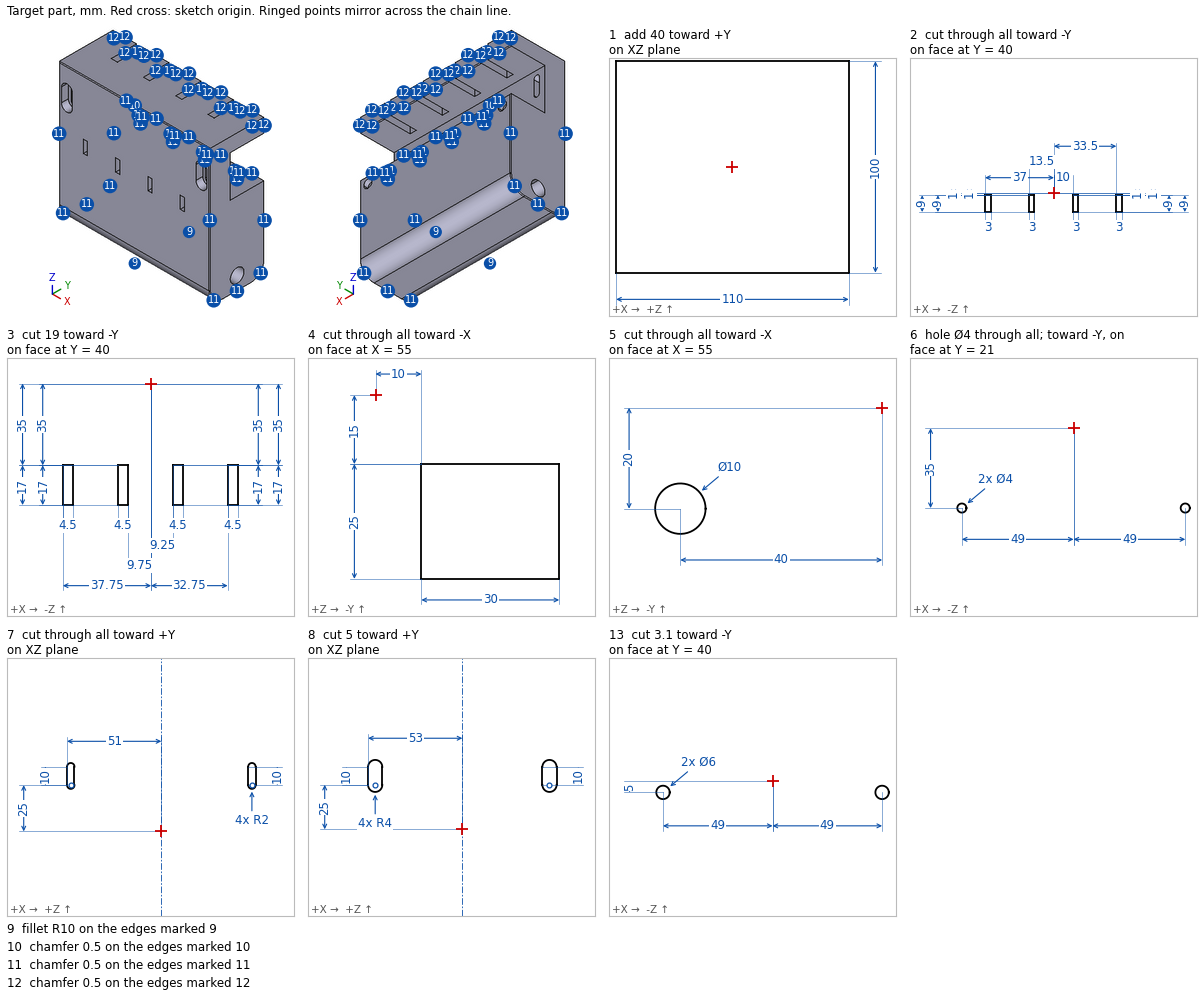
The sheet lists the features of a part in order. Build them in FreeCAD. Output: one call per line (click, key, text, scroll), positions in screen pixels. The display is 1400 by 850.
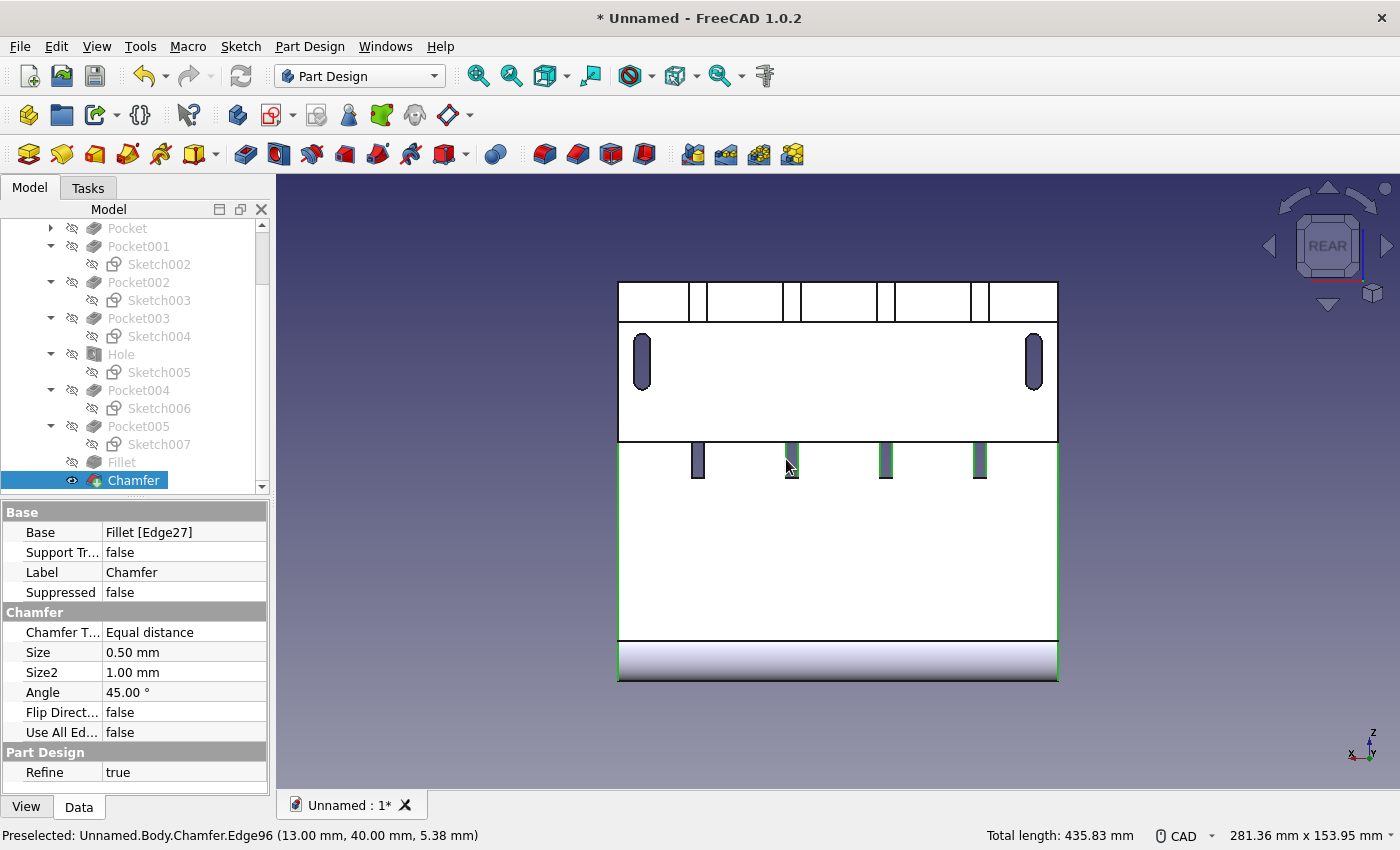
click(704, 459, ctrl)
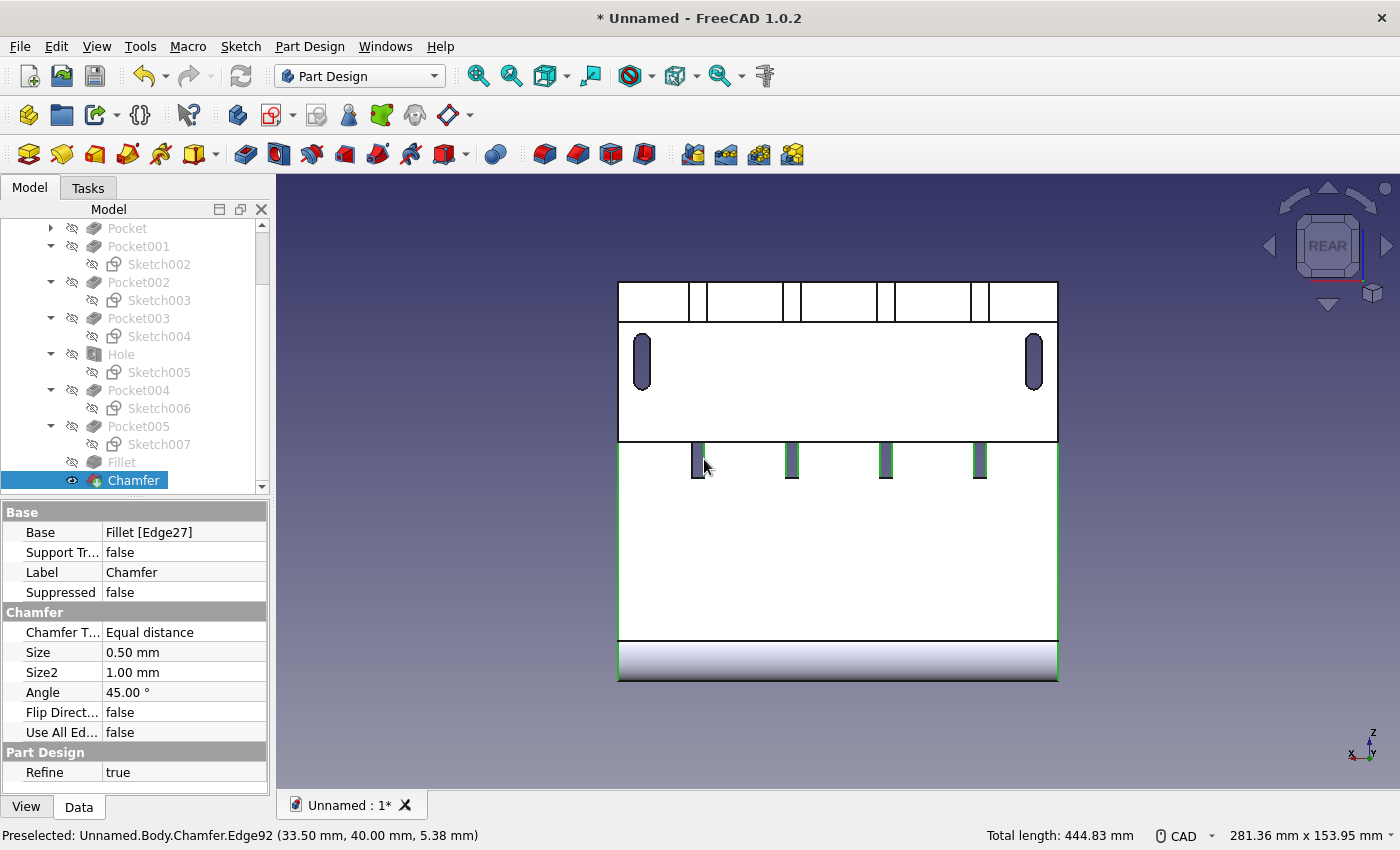
click(692, 459, ctrl)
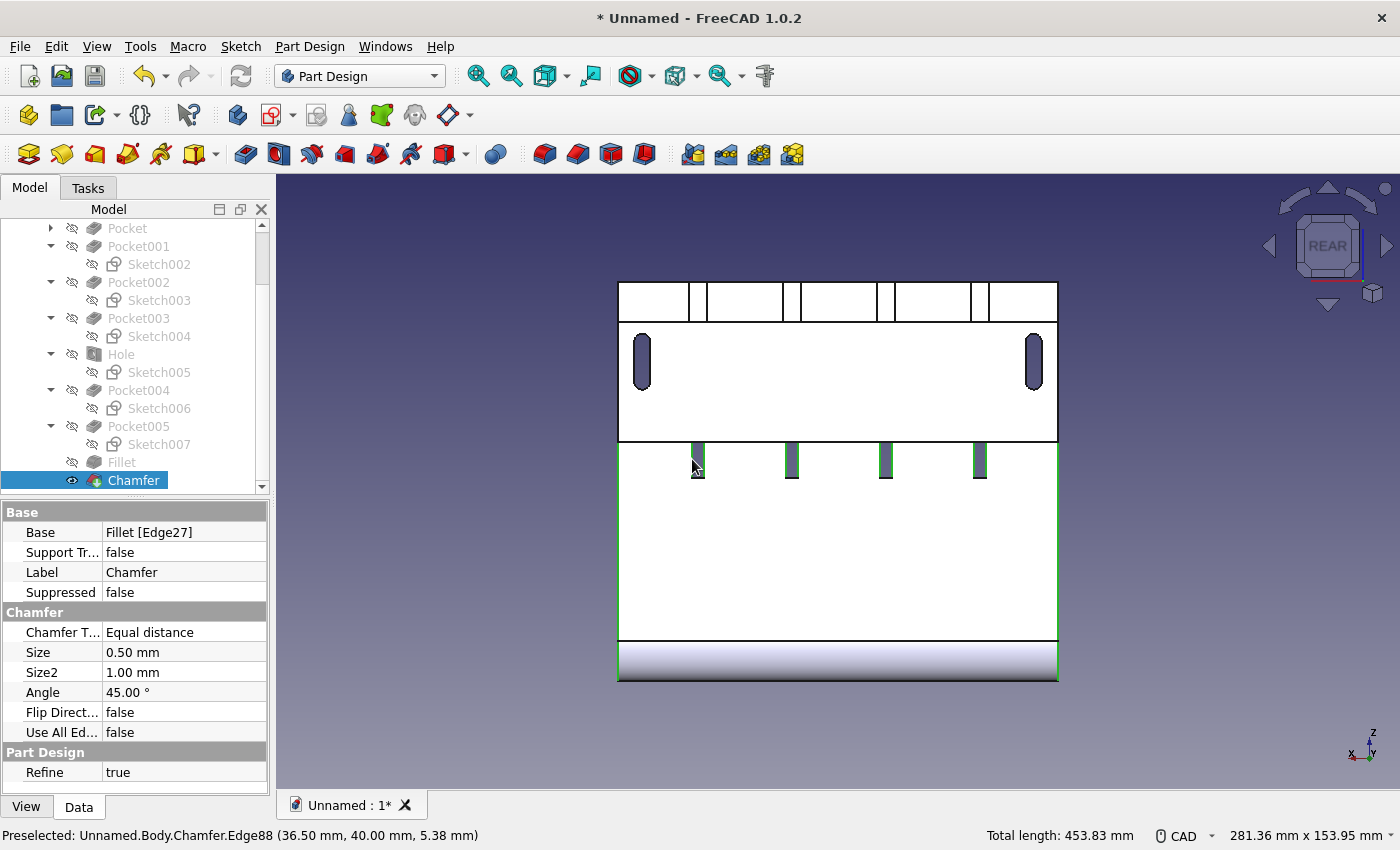
key(6)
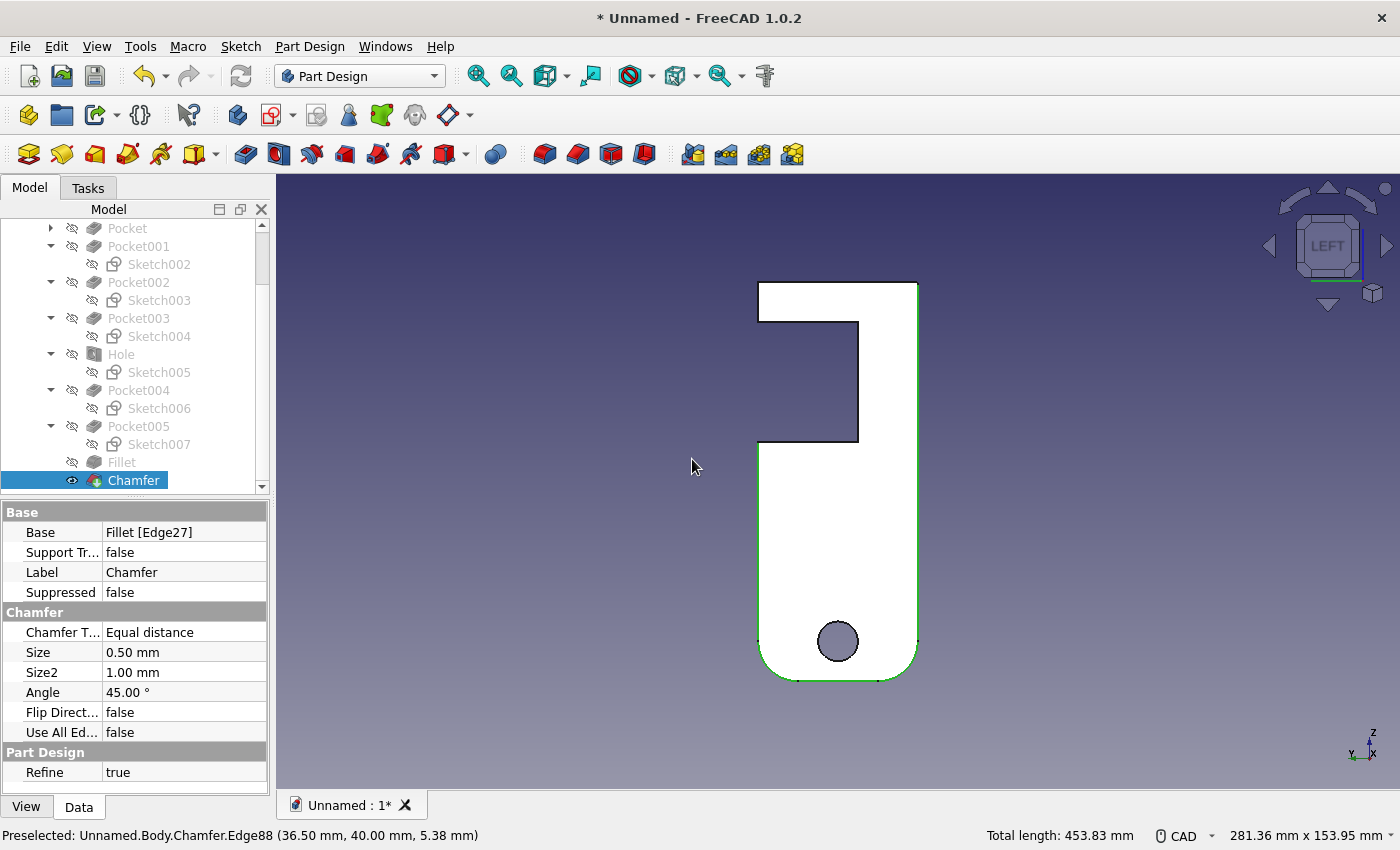
key(v)
key(3)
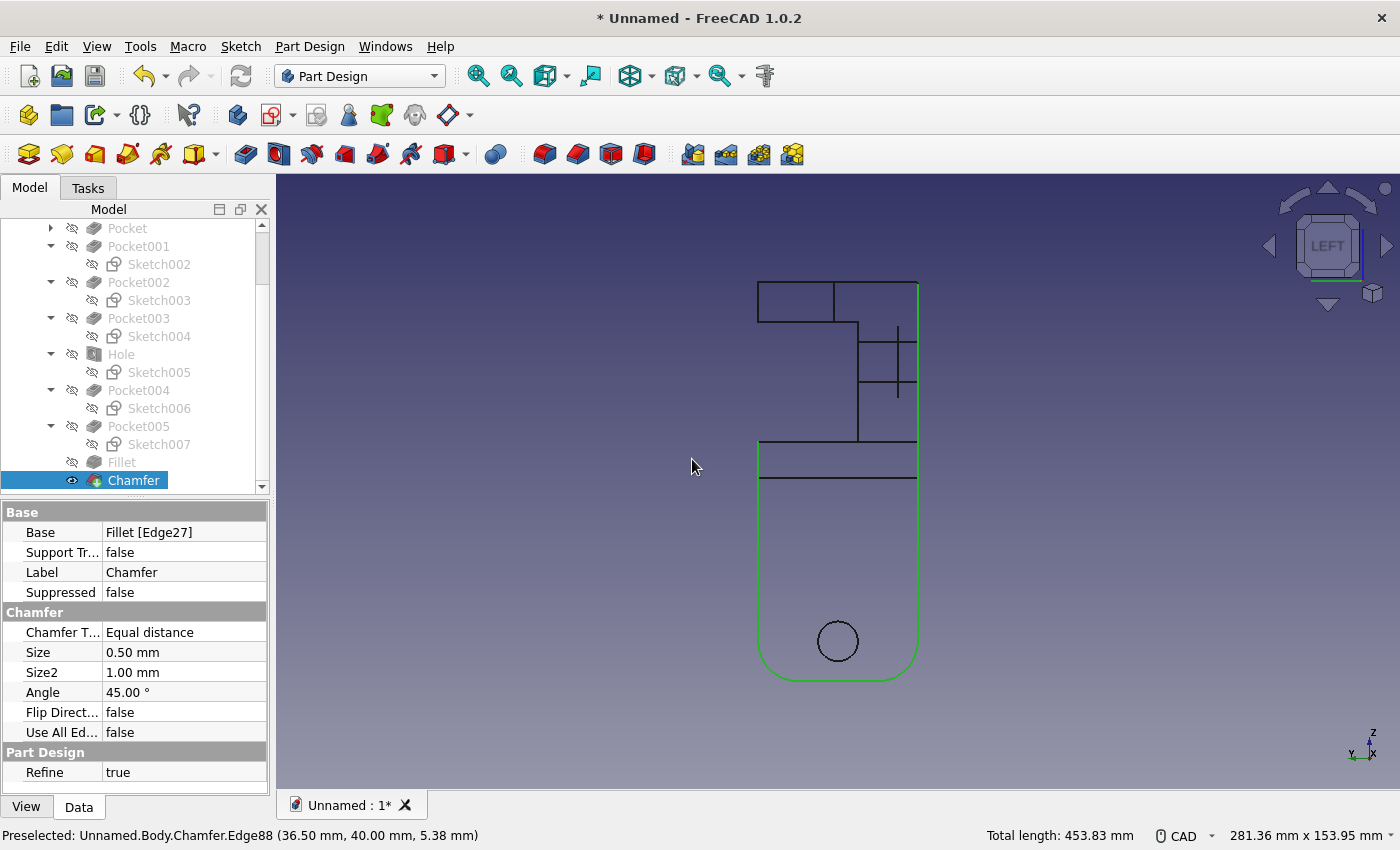
key(0)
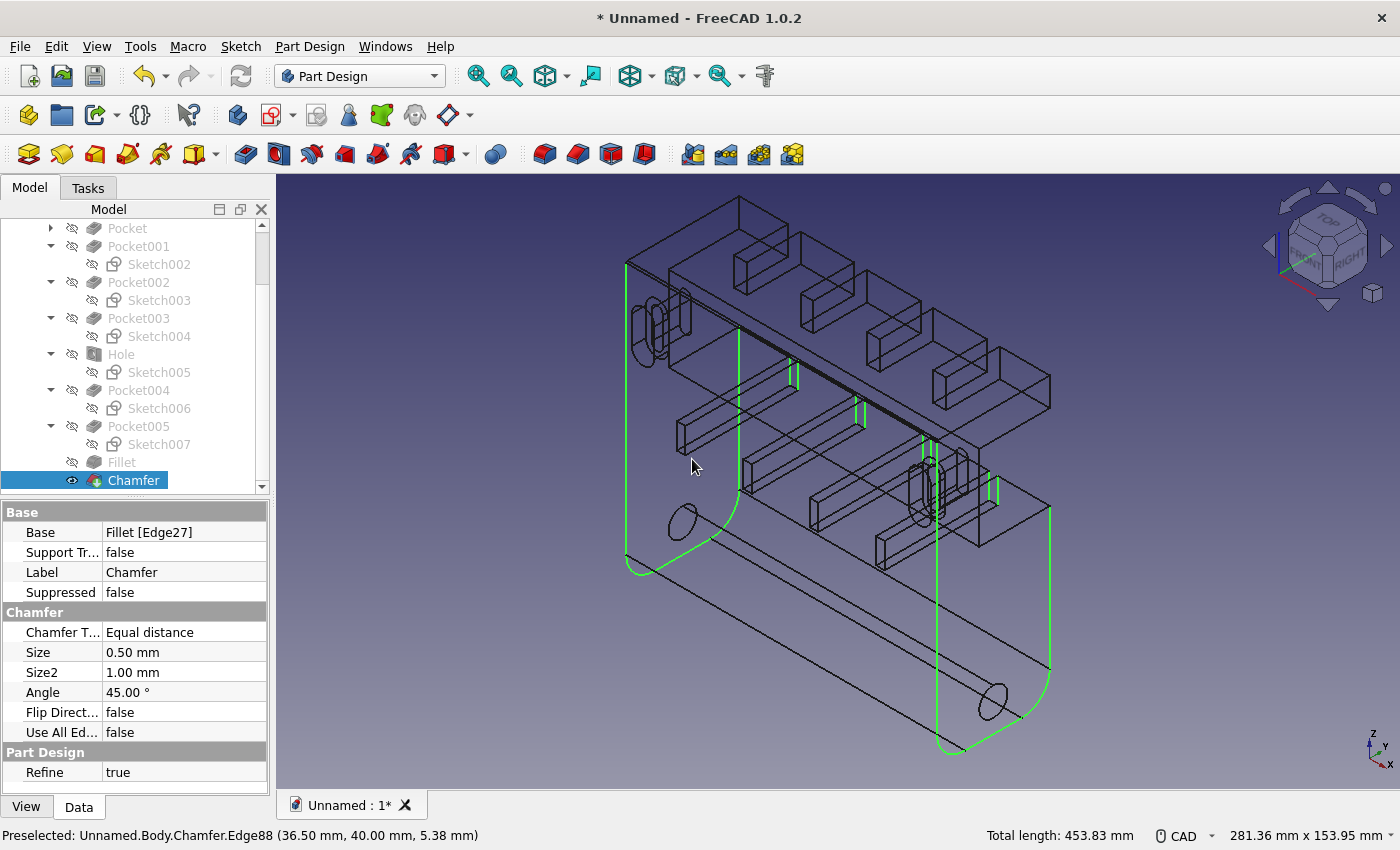
click(792, 385, ctrl)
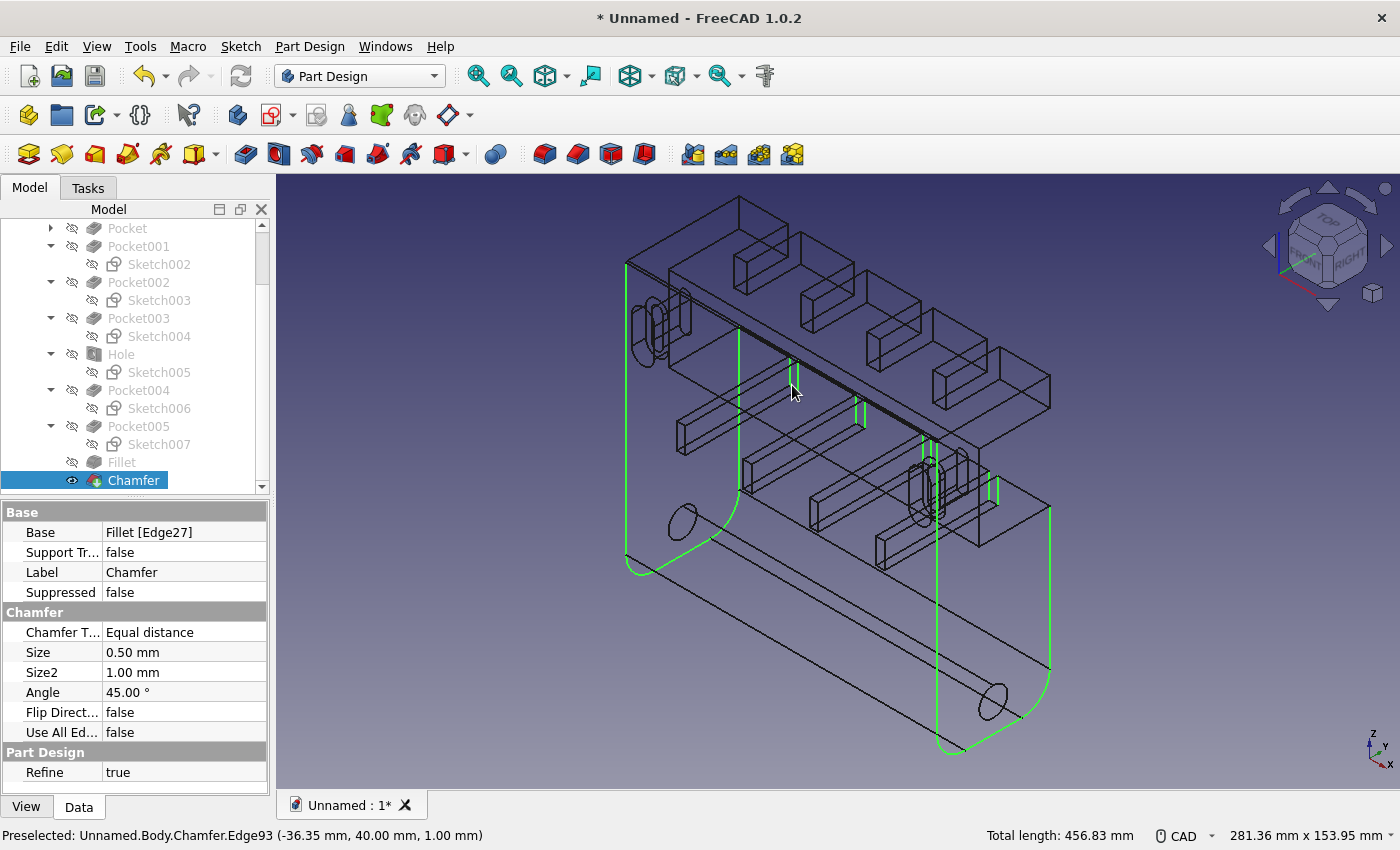
click(858, 424, ctrl)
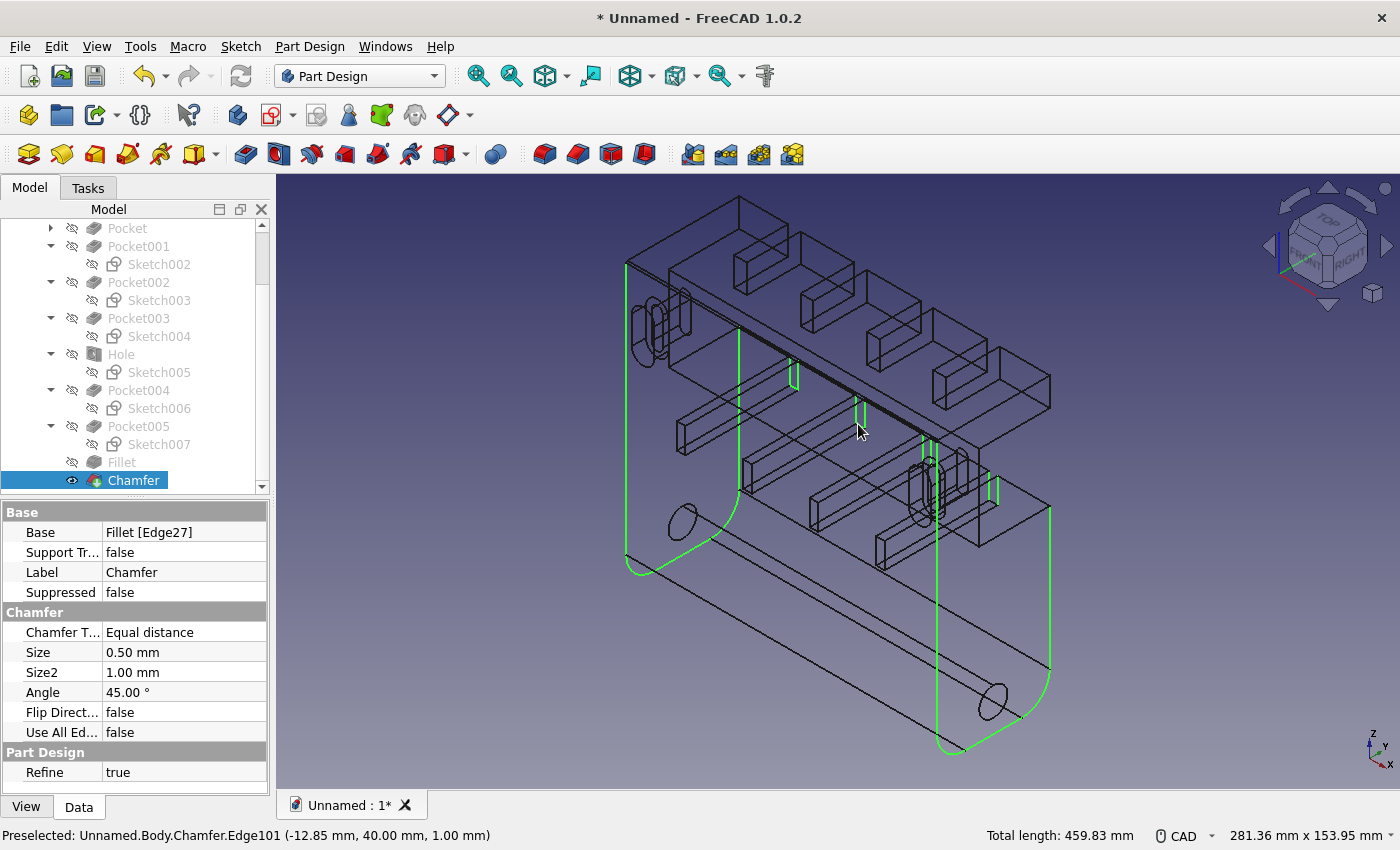
click(949, 446, ctrl)